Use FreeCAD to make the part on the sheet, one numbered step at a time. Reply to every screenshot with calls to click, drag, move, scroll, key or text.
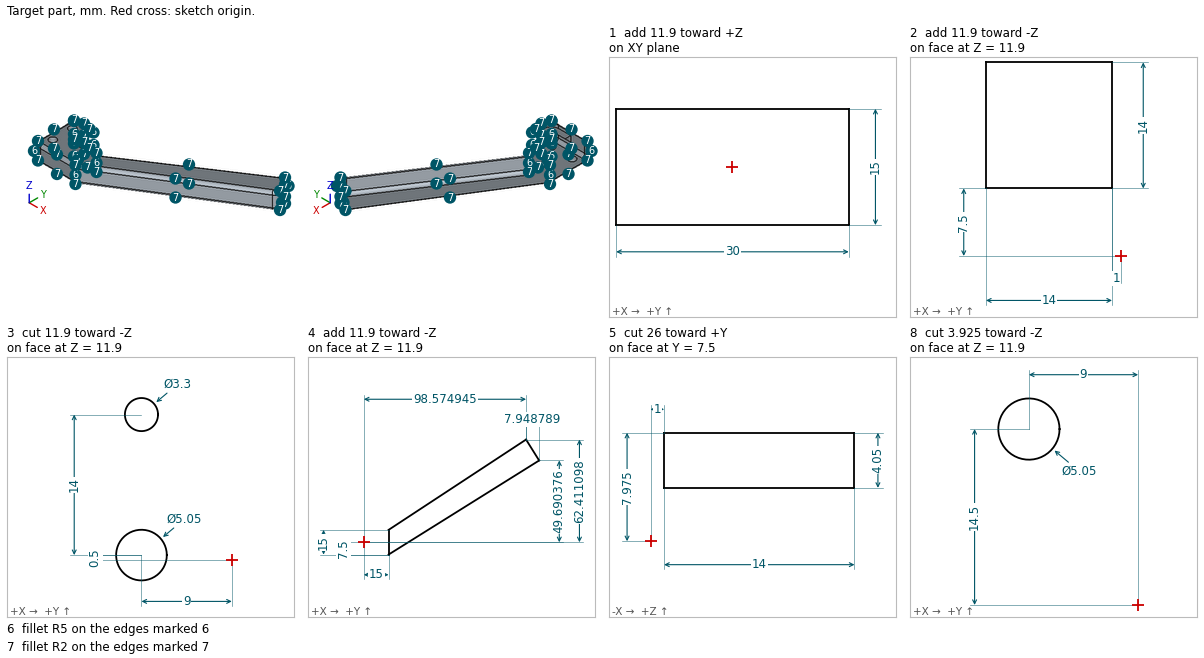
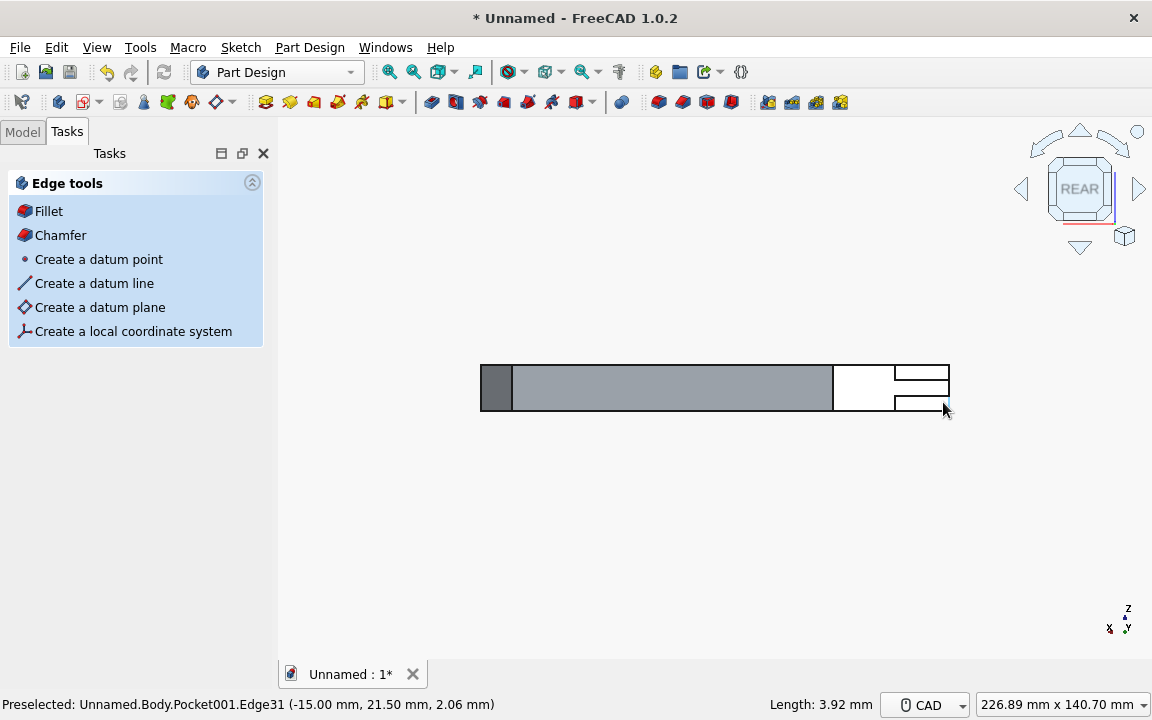
click(512, 387, ctrl)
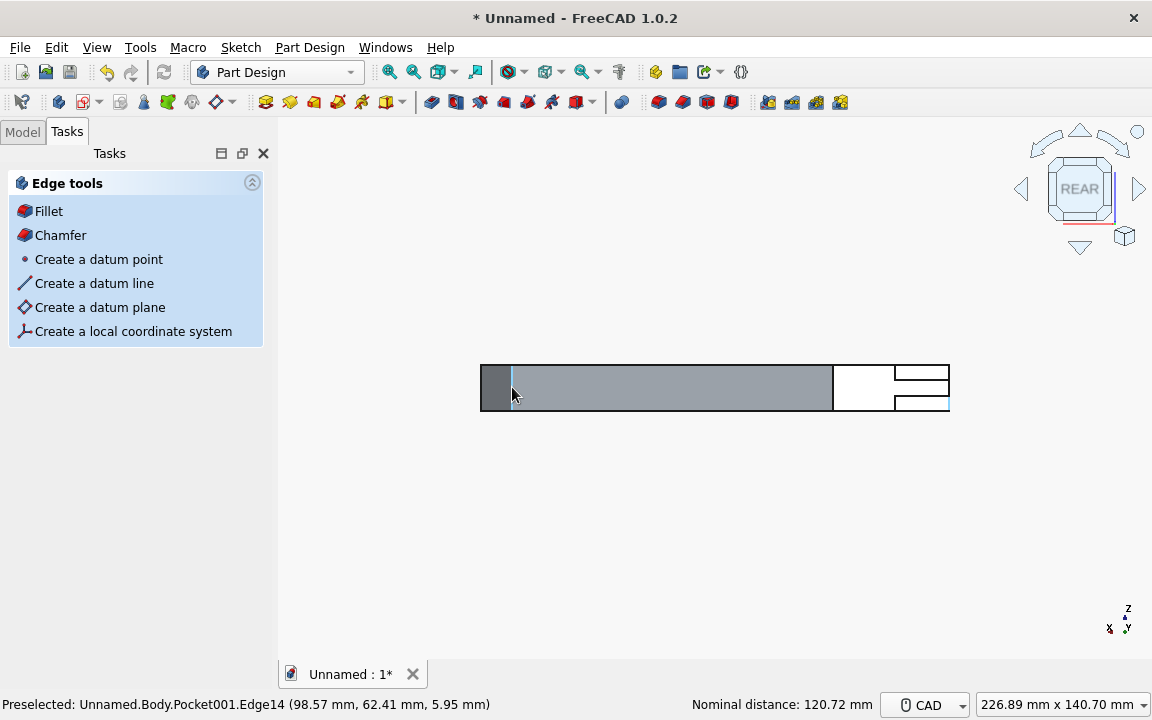
click(949, 372, ctrl)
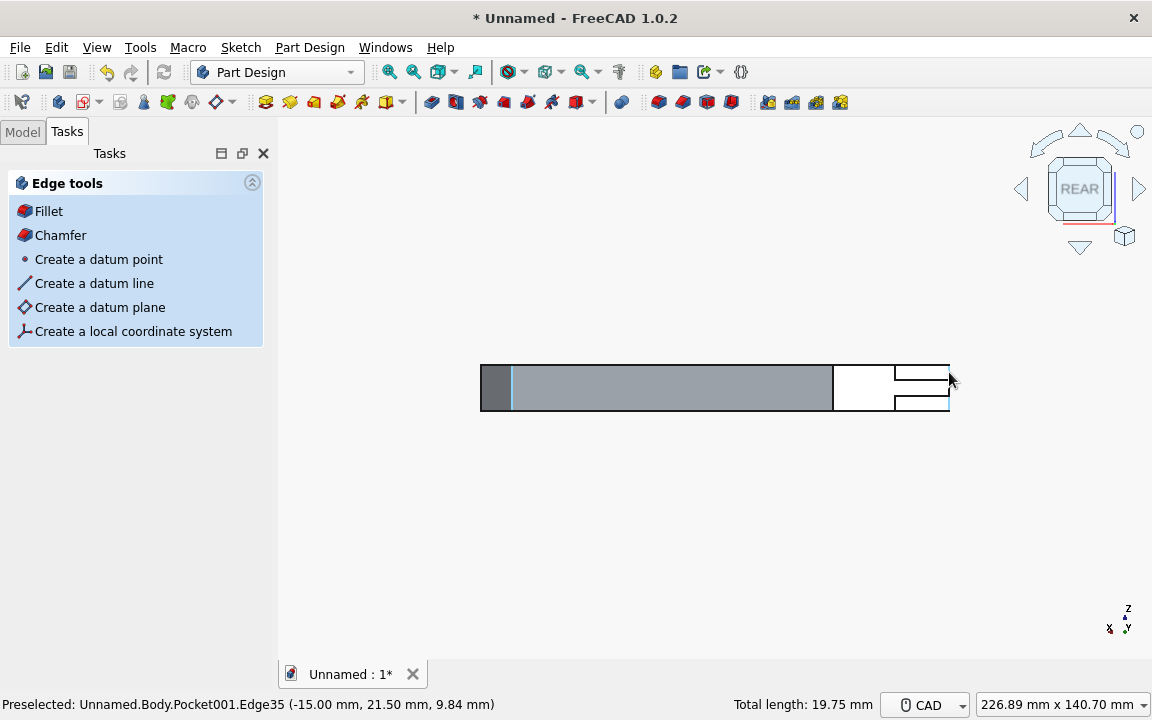
scroll(895, 402, up, 5)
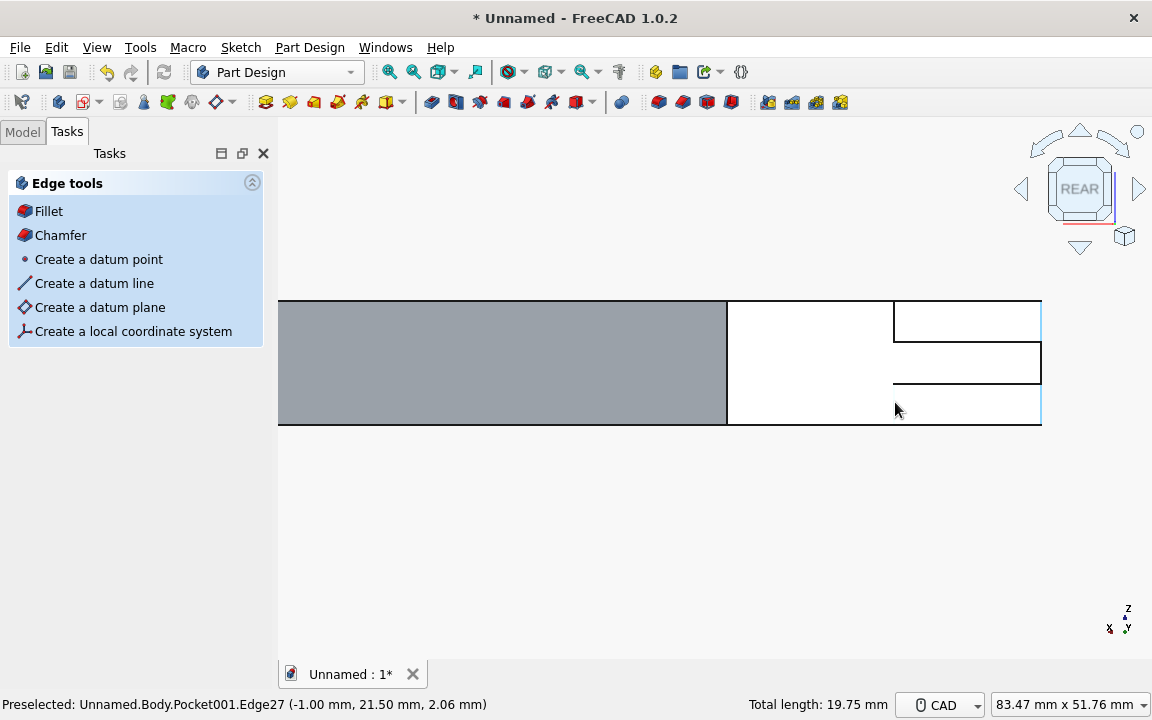
click(390, 72)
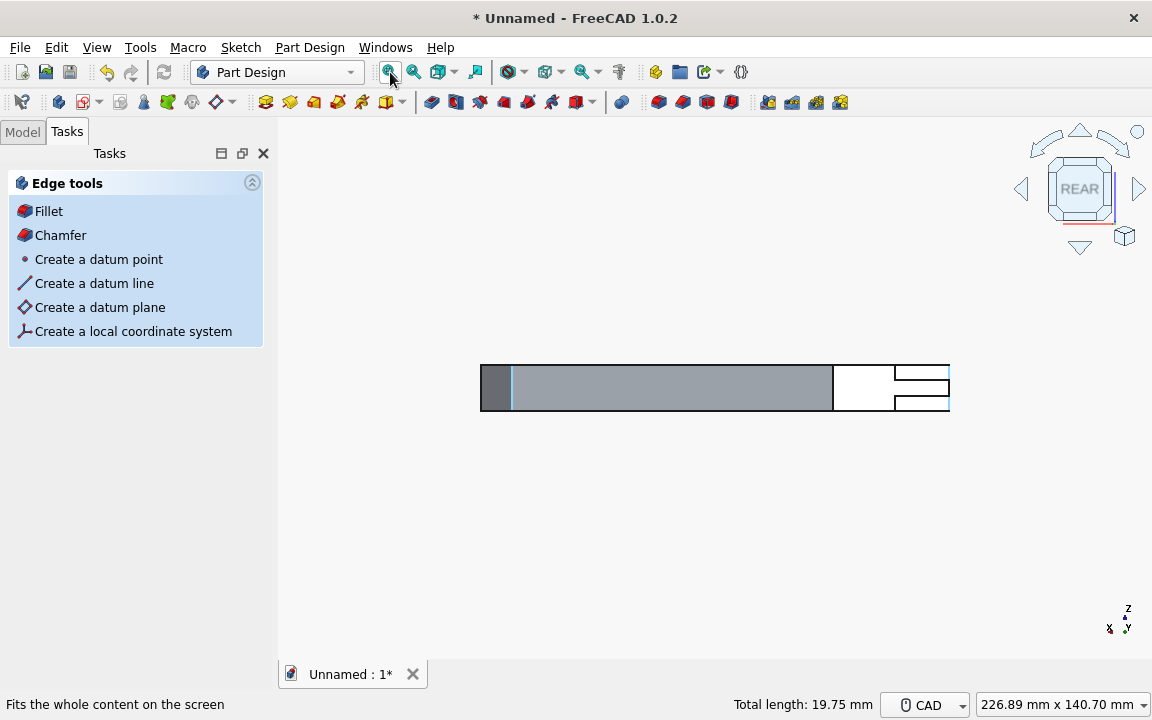
key(0)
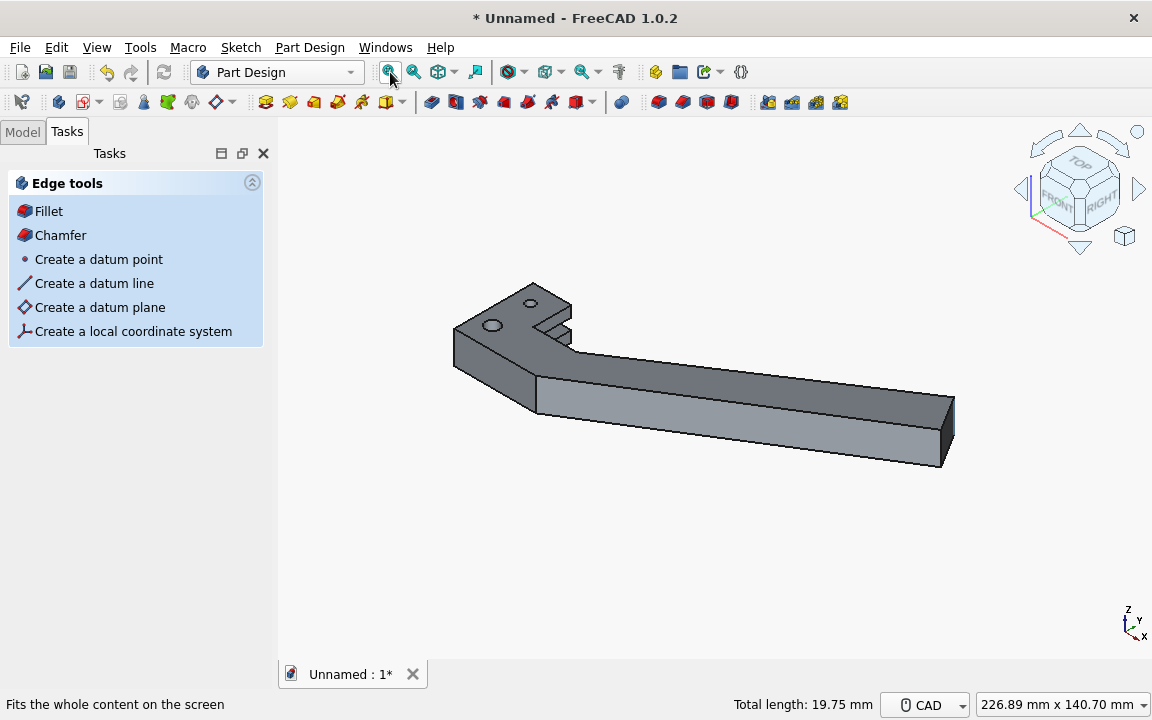
click(941, 448, ctrl)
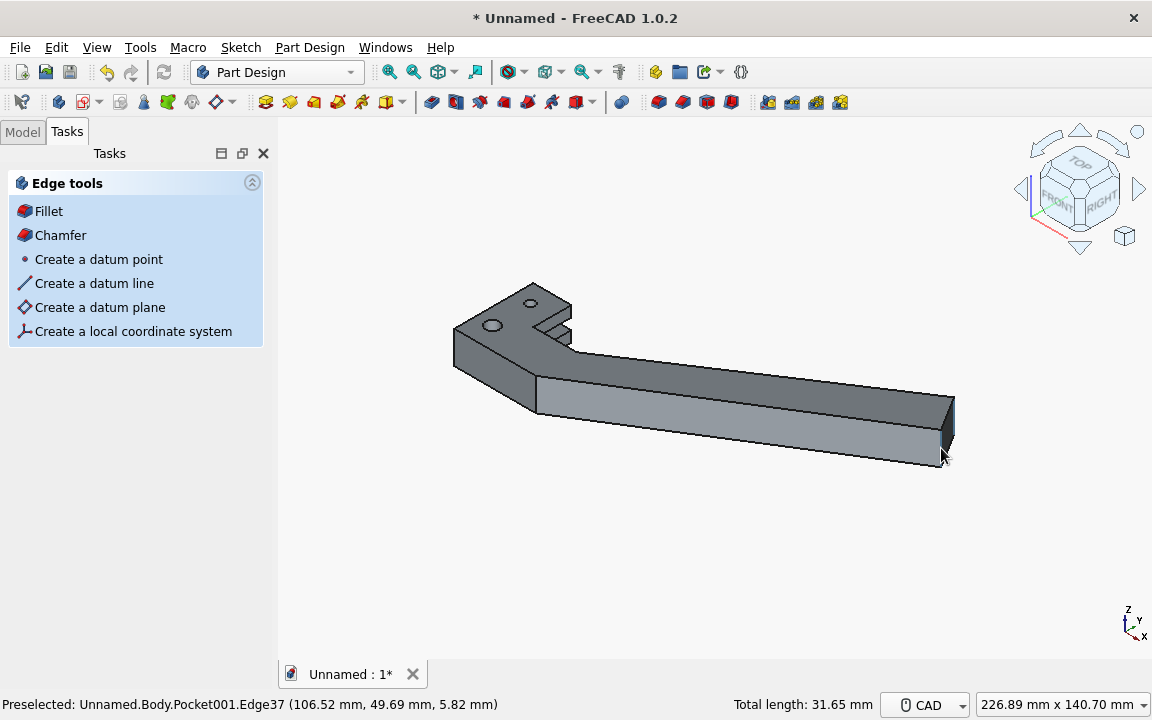
scroll(571, 335, up, 5)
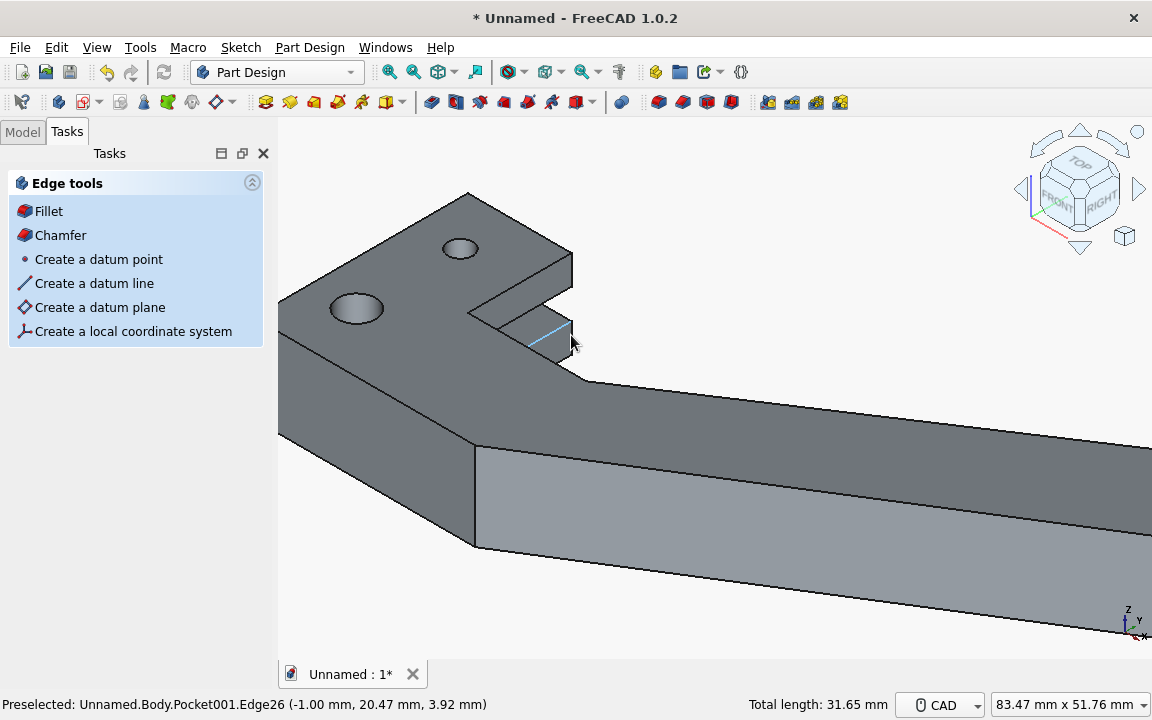
click(390, 72)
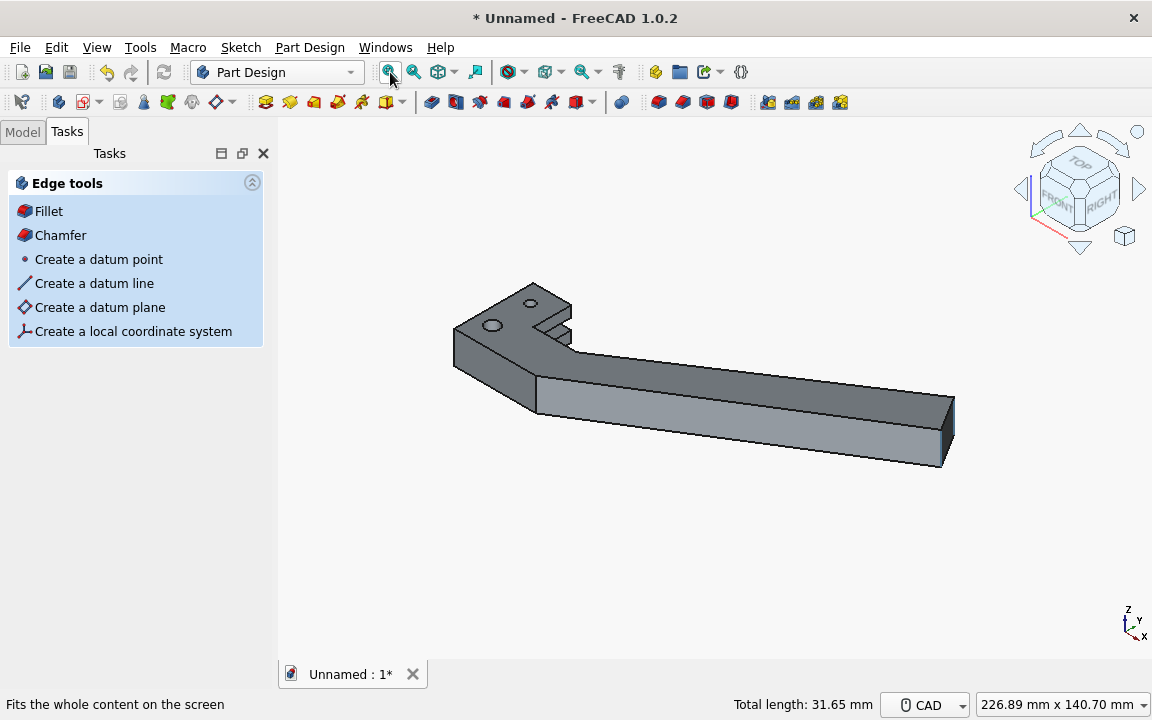
key(2)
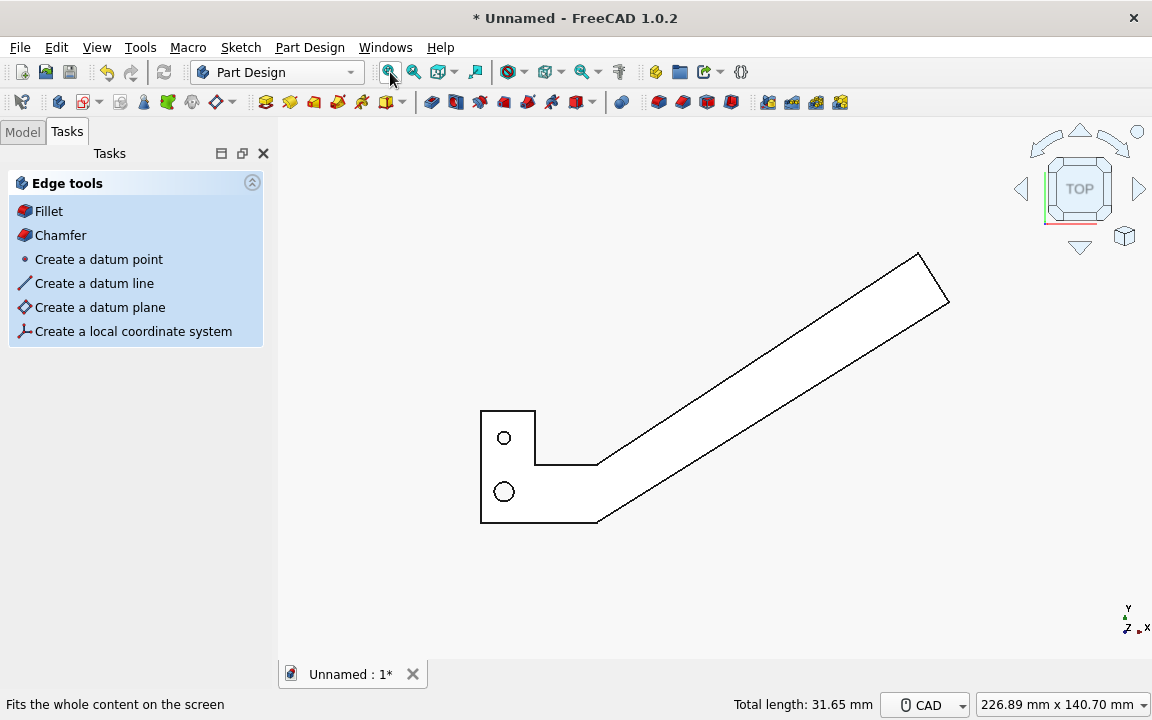
scroll(535, 410, up, 5)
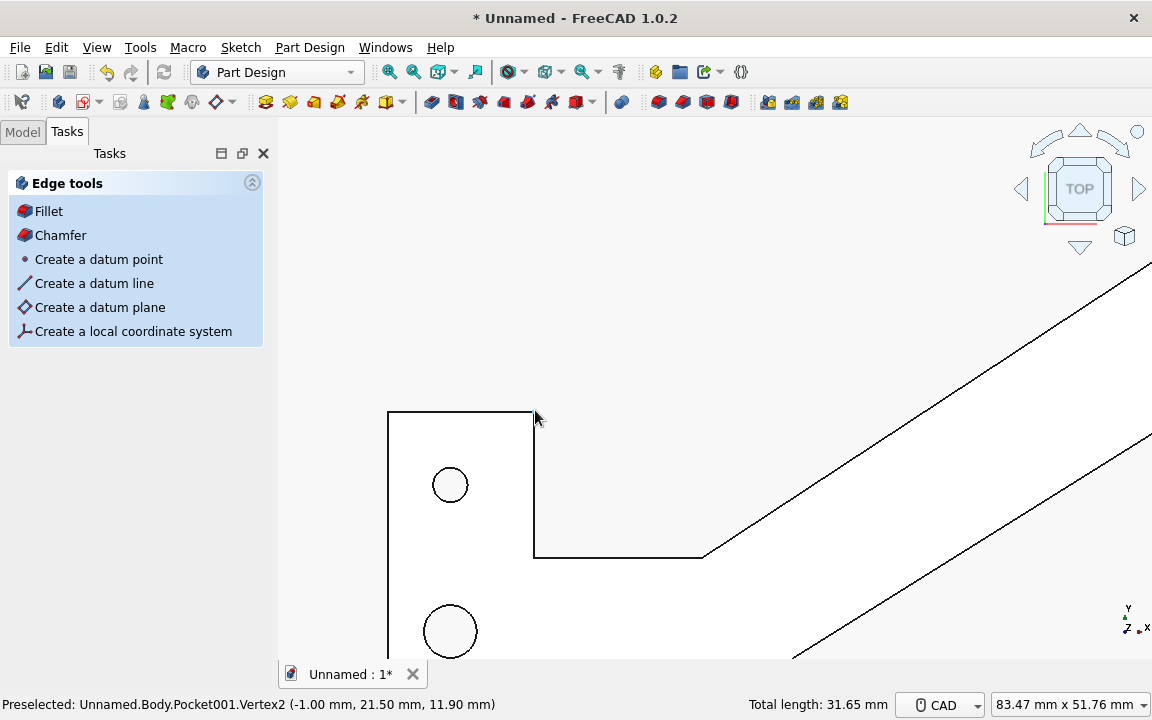
click(390, 72)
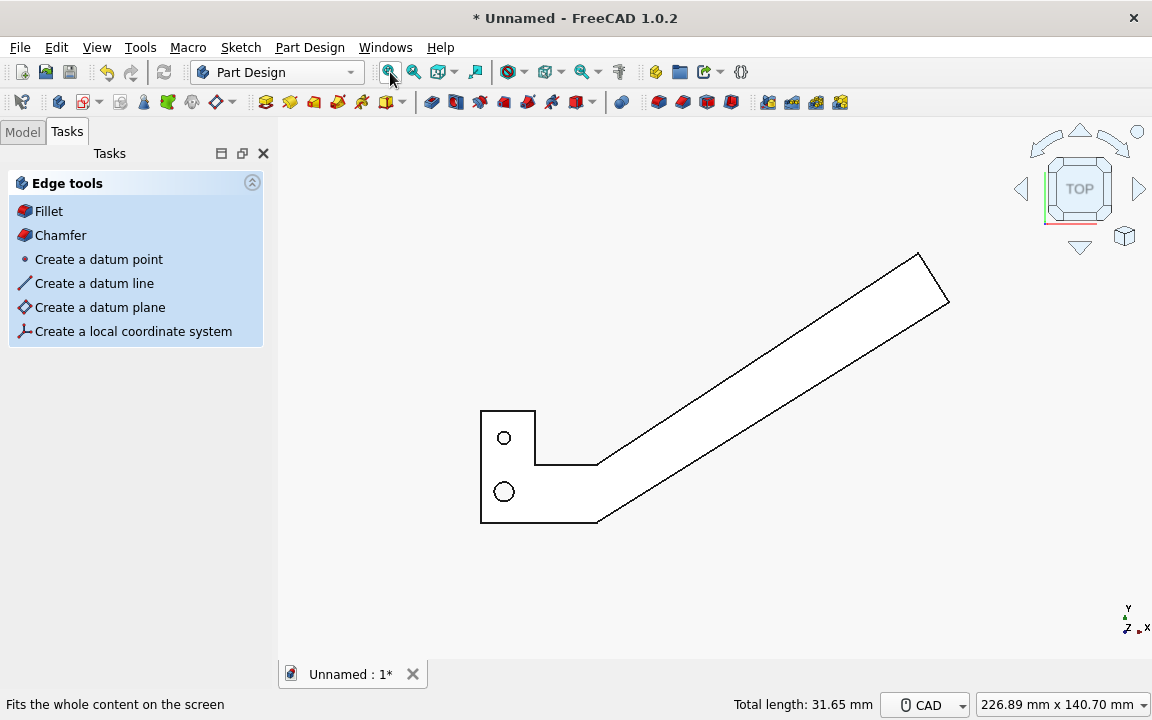
key(1)